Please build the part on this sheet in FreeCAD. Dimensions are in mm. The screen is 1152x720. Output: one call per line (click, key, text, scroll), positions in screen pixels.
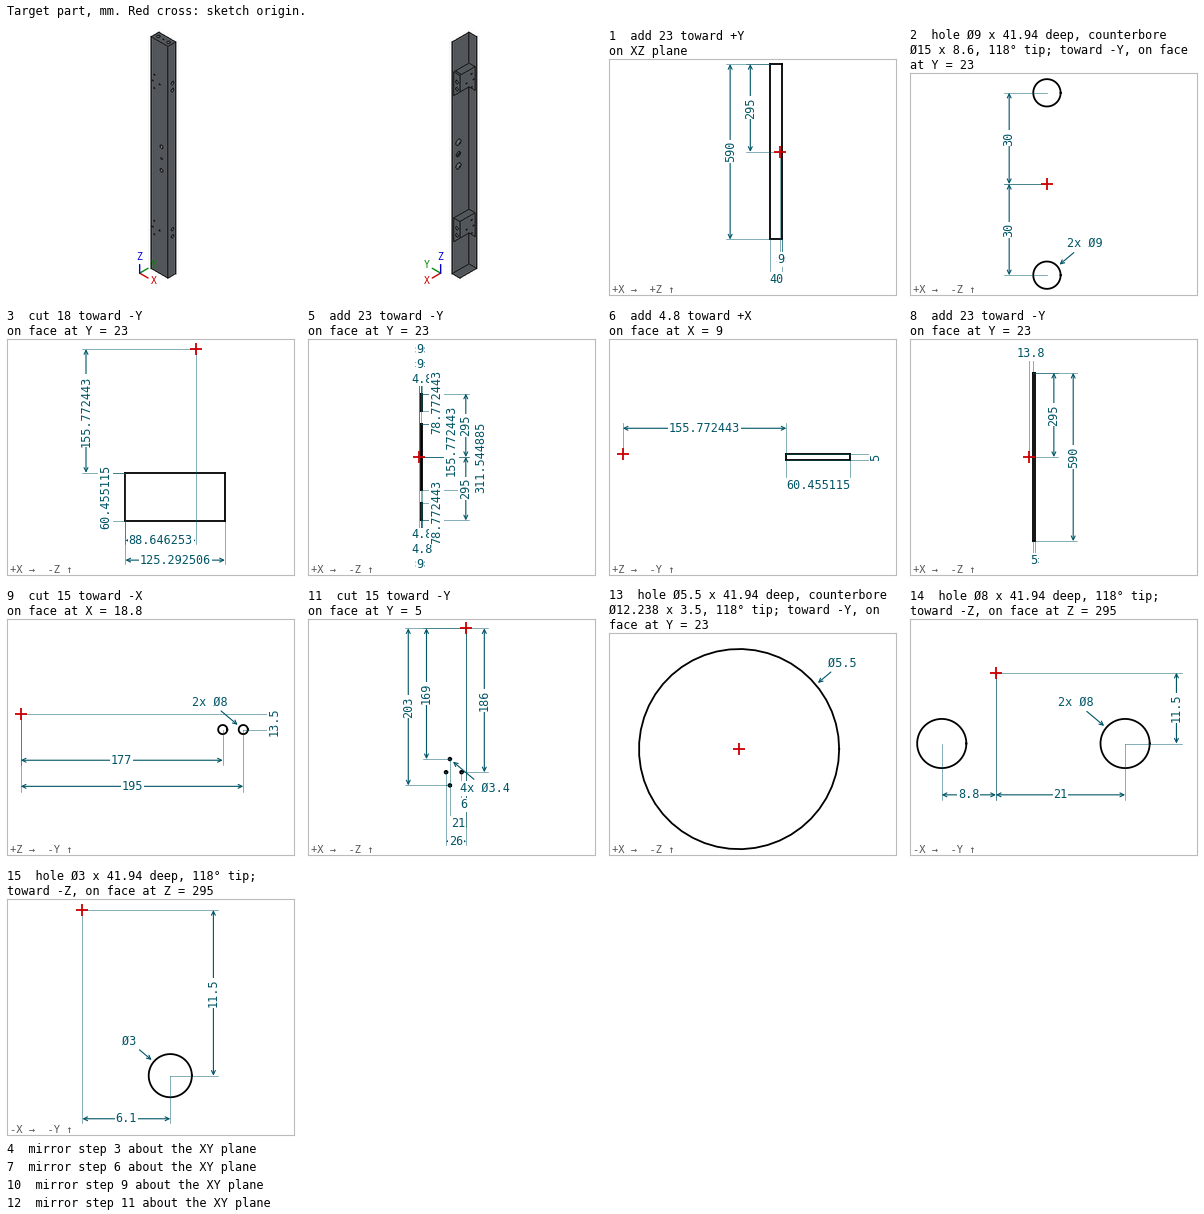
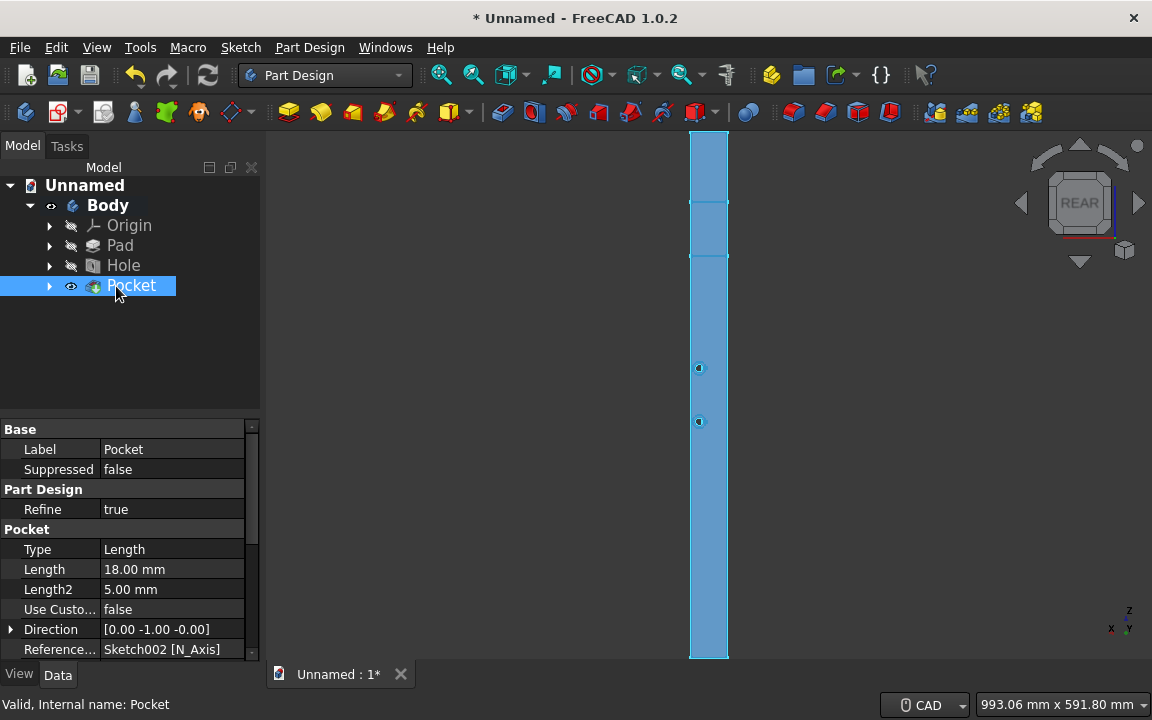
click(936, 112)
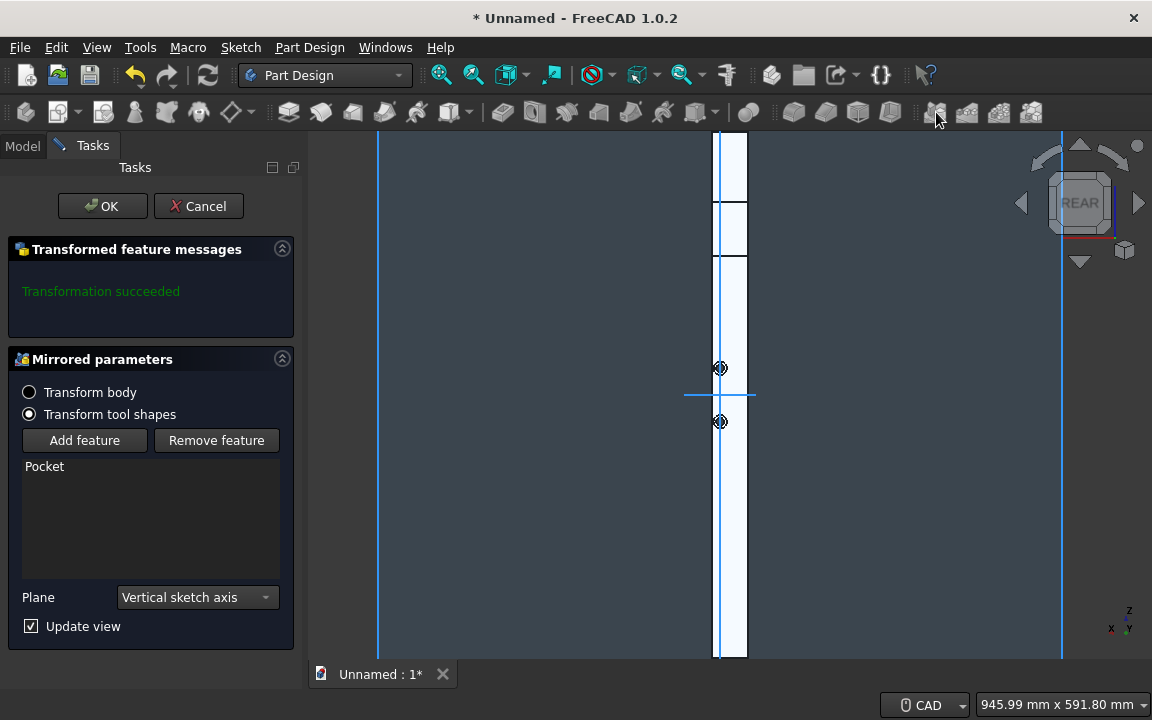
click(198, 598)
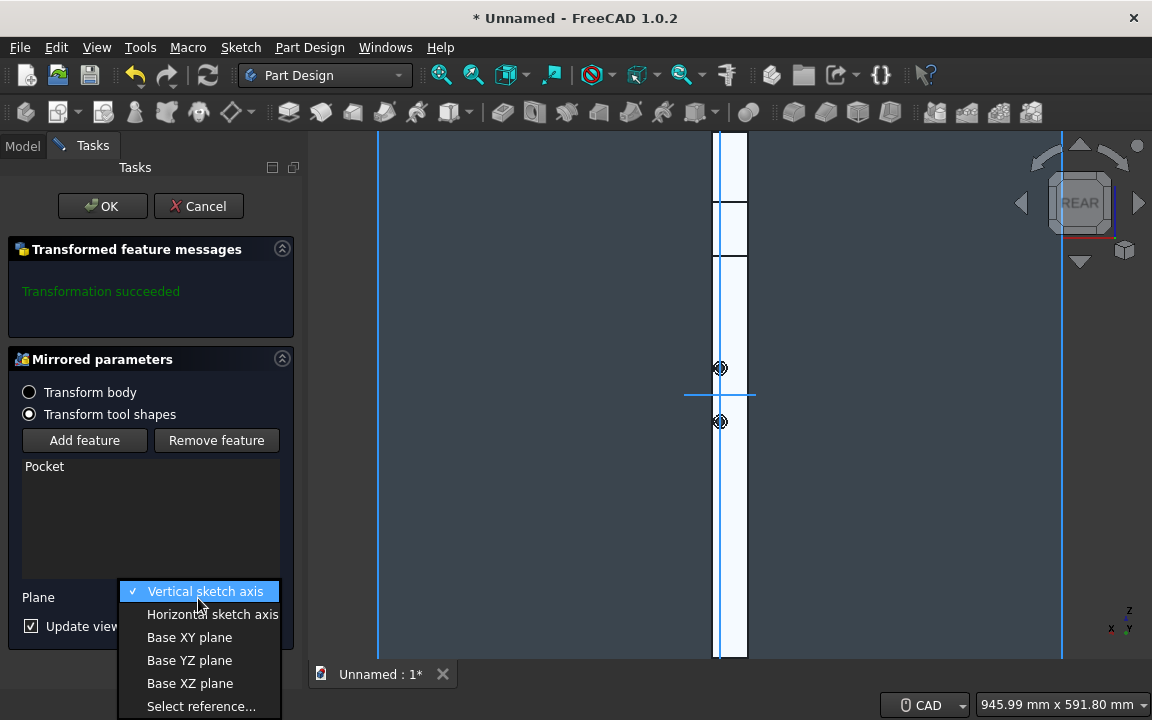
click(198, 638)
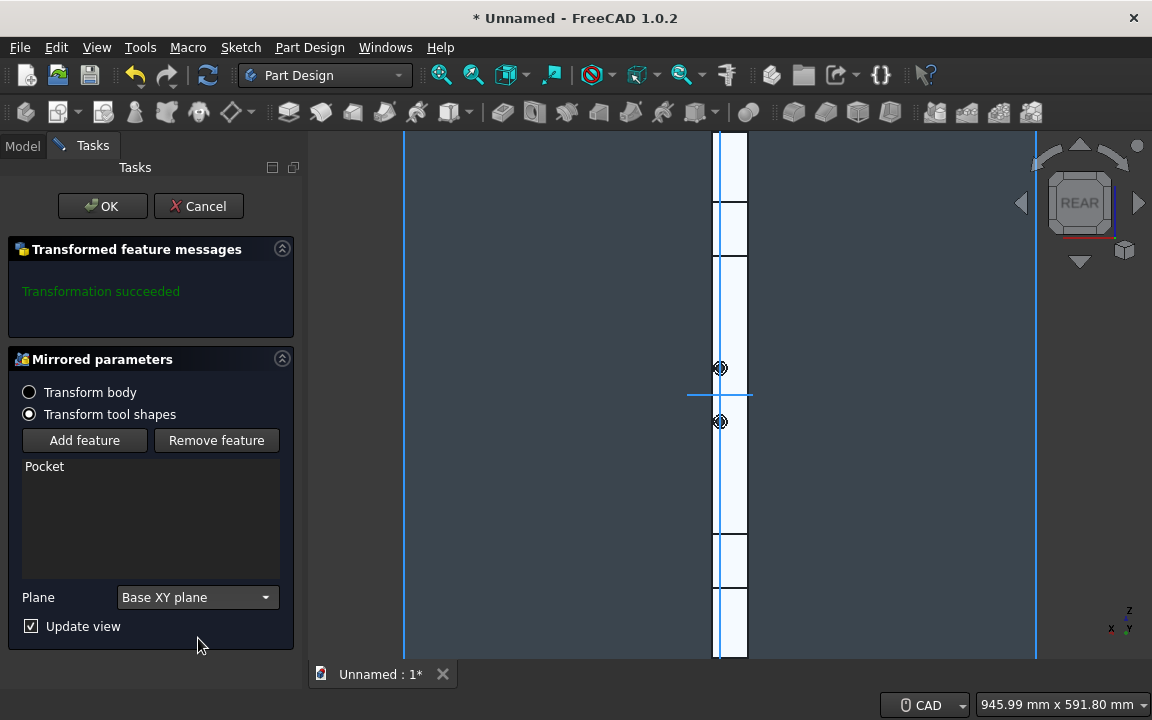
click(103, 206)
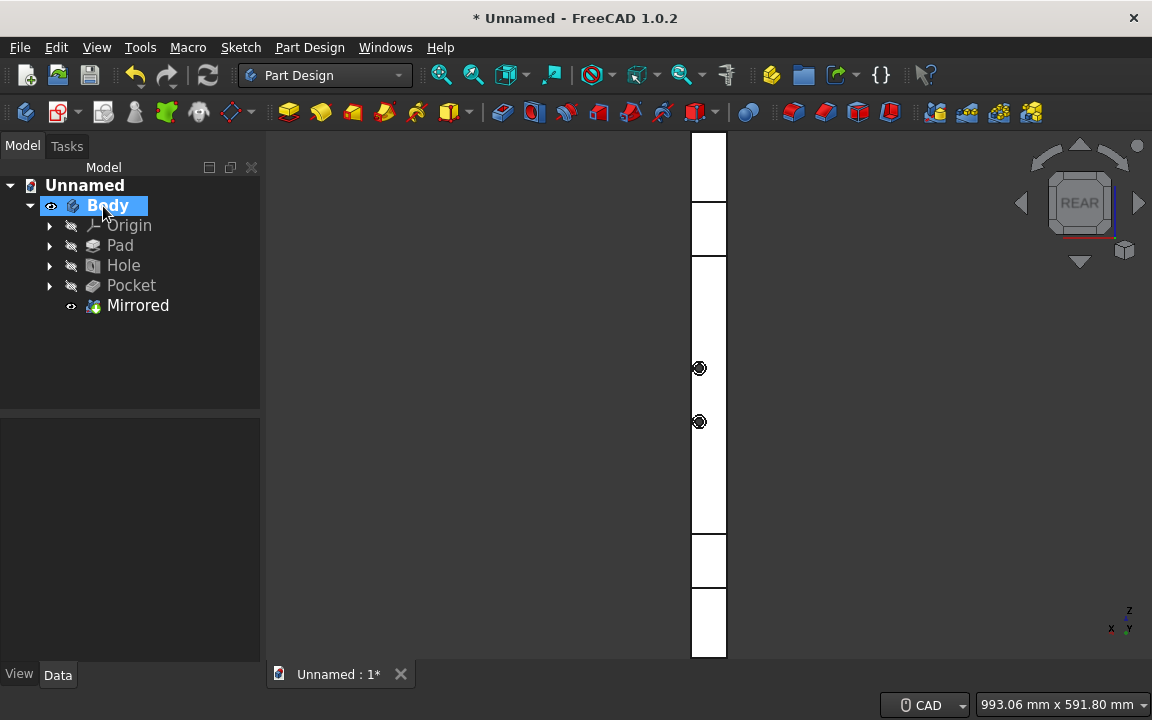
click(709, 275)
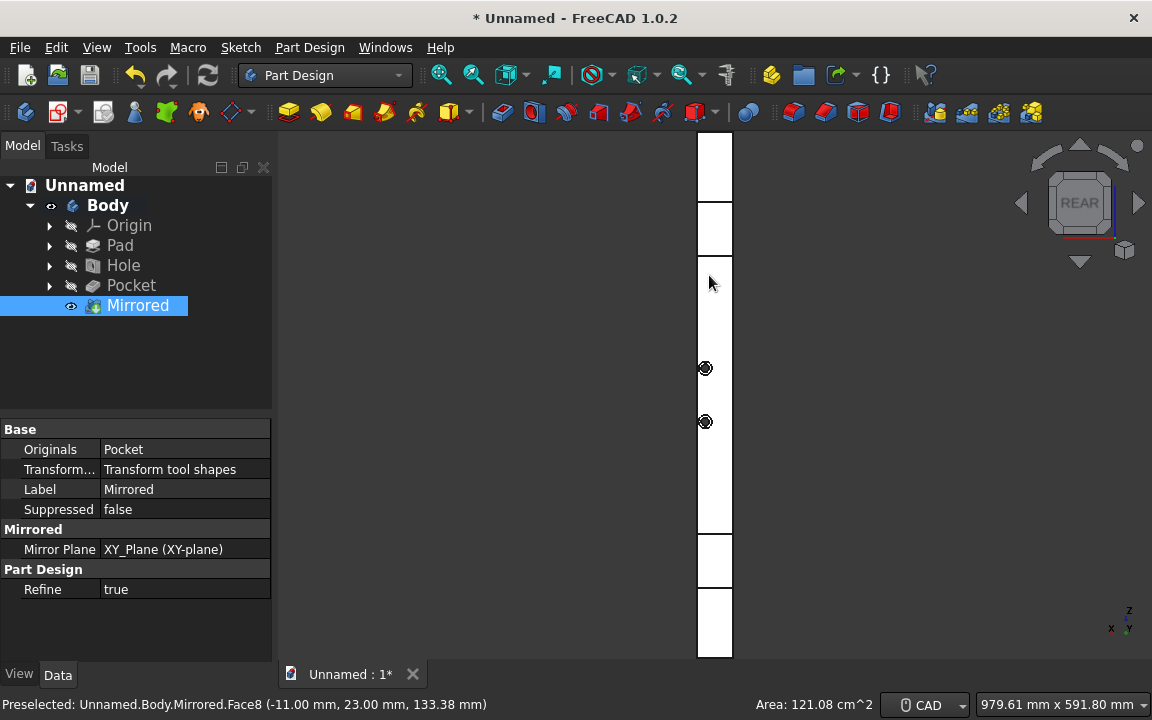
click(58, 112)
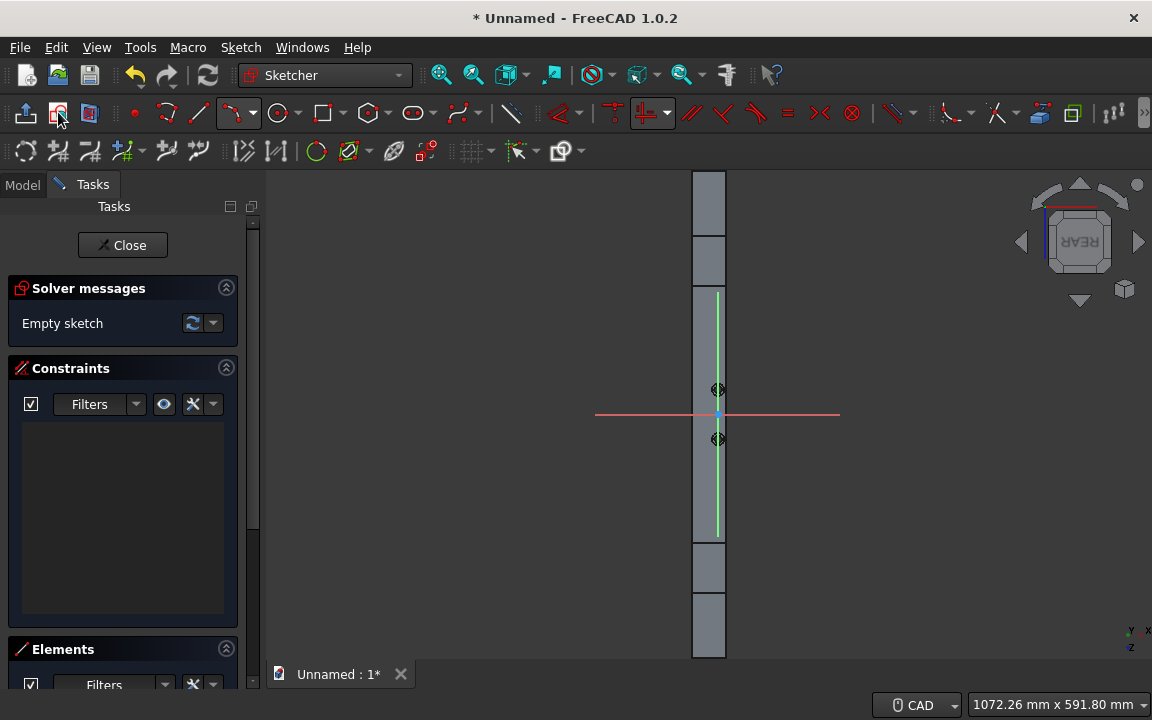
scroll(471, 415, down, 2)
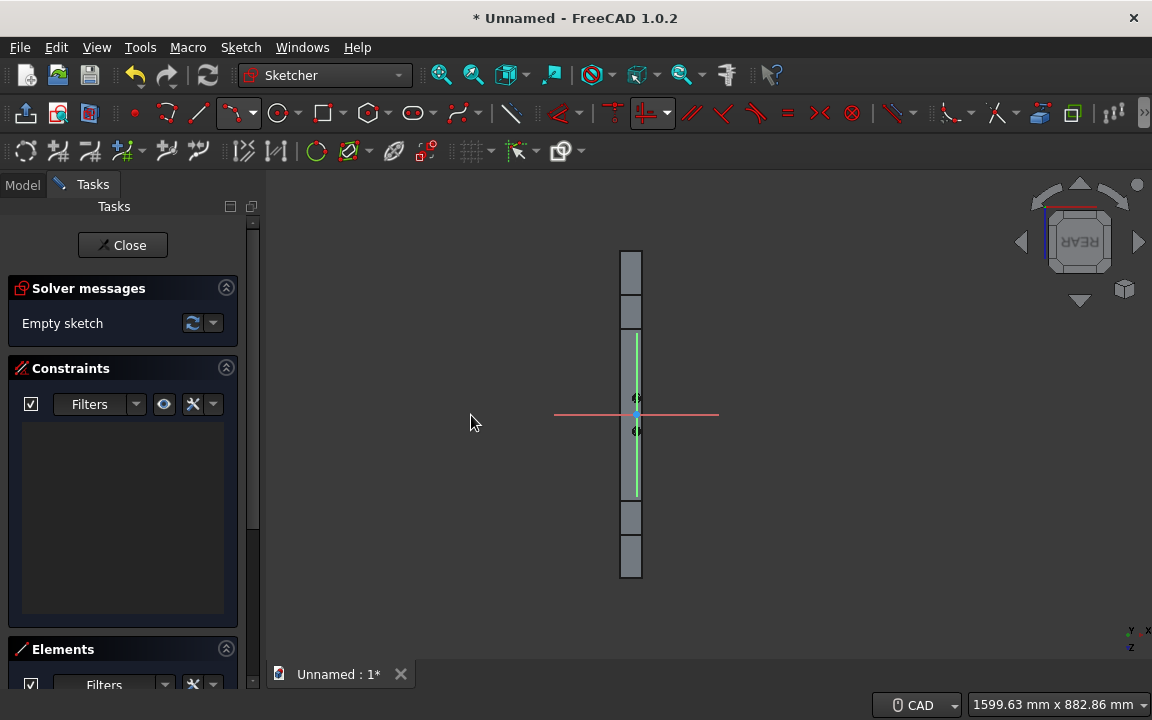
click(324, 114)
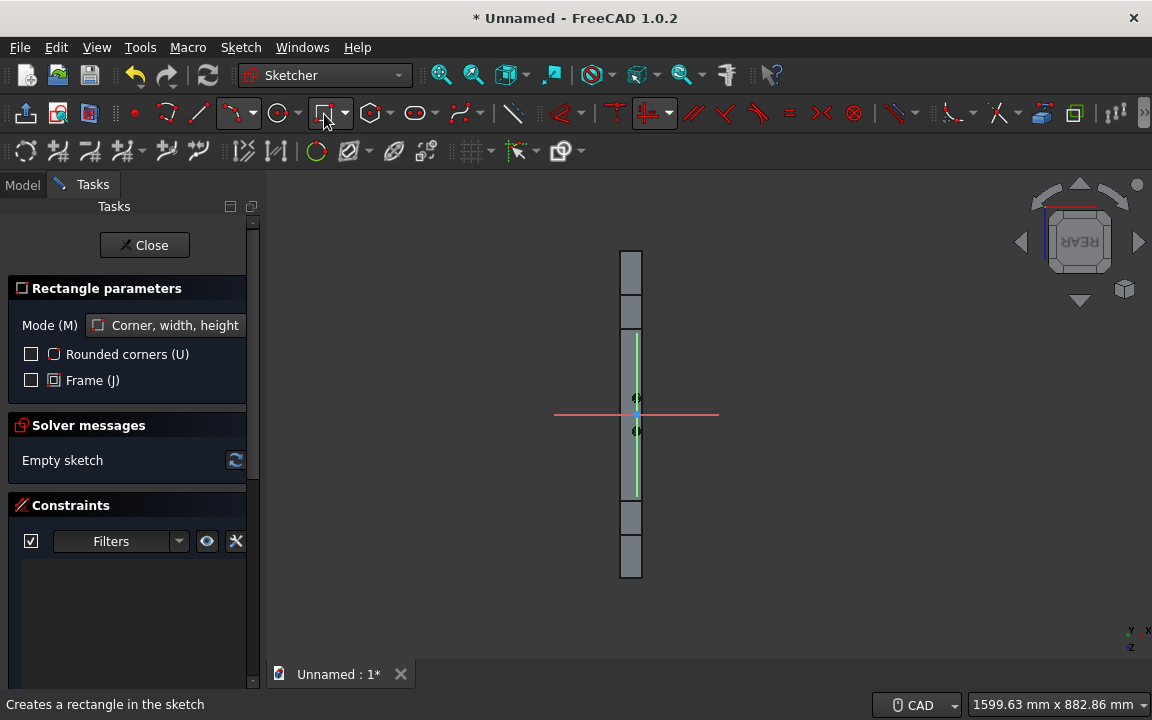
scroll(642, 535, up, 9)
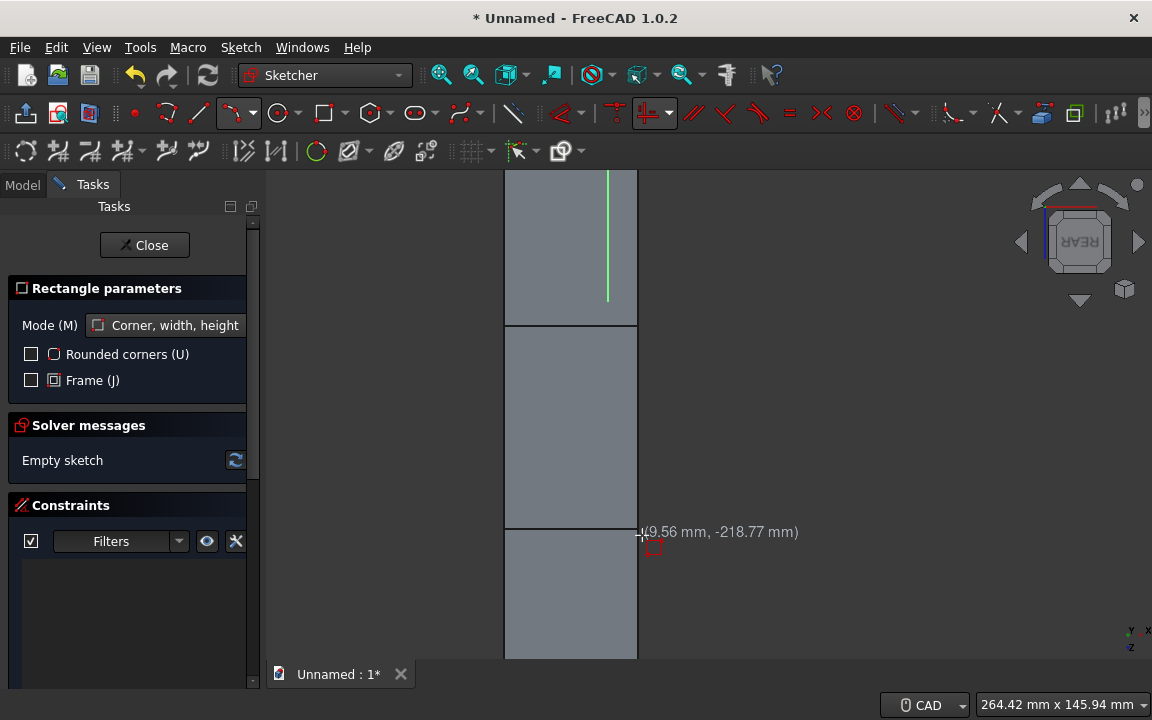
click(638, 529)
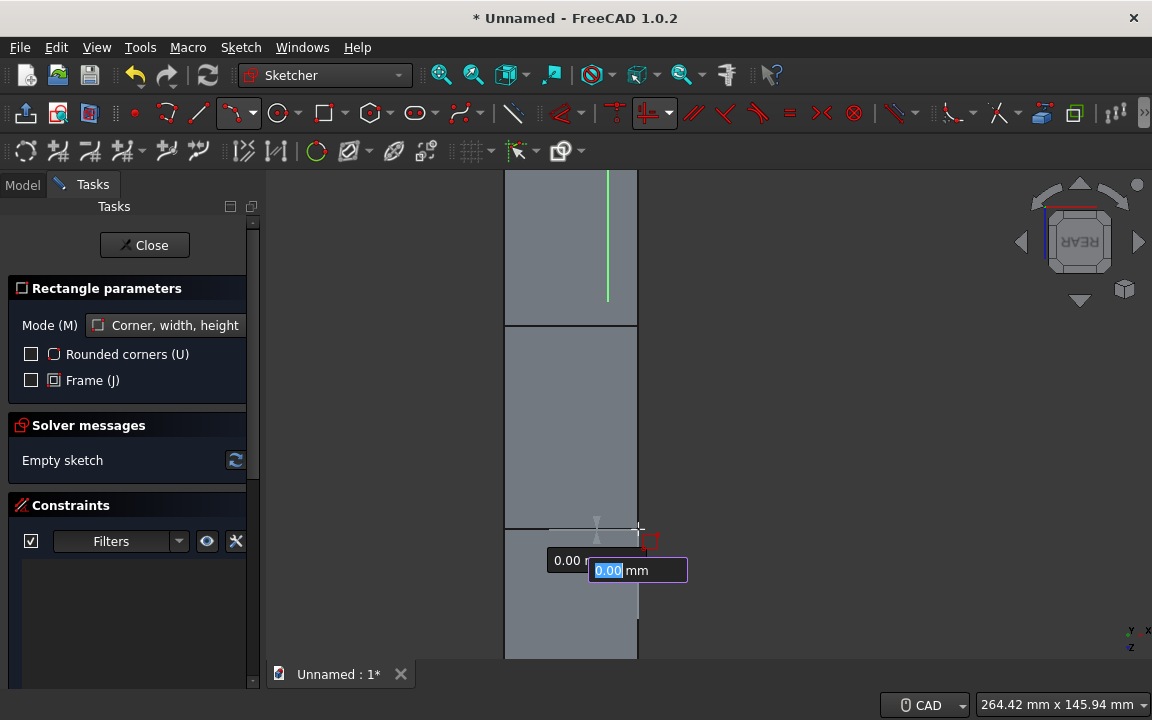
scroll(642, 535, down, 9)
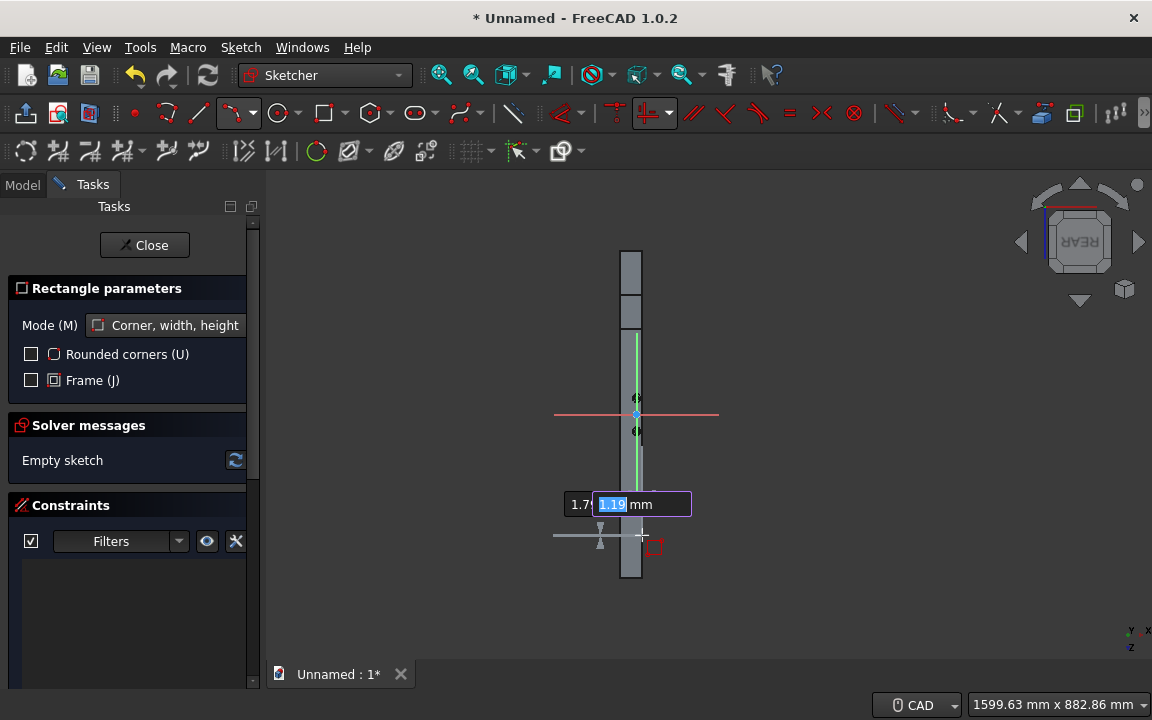
scroll(644, 578, up, 4)